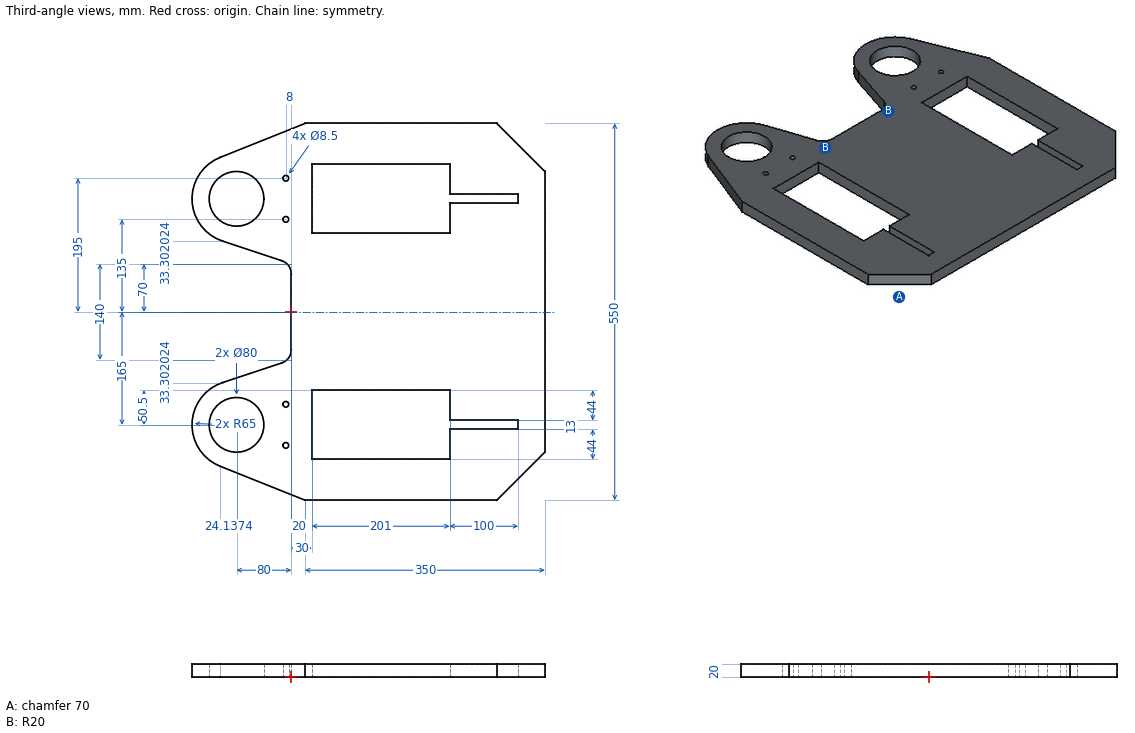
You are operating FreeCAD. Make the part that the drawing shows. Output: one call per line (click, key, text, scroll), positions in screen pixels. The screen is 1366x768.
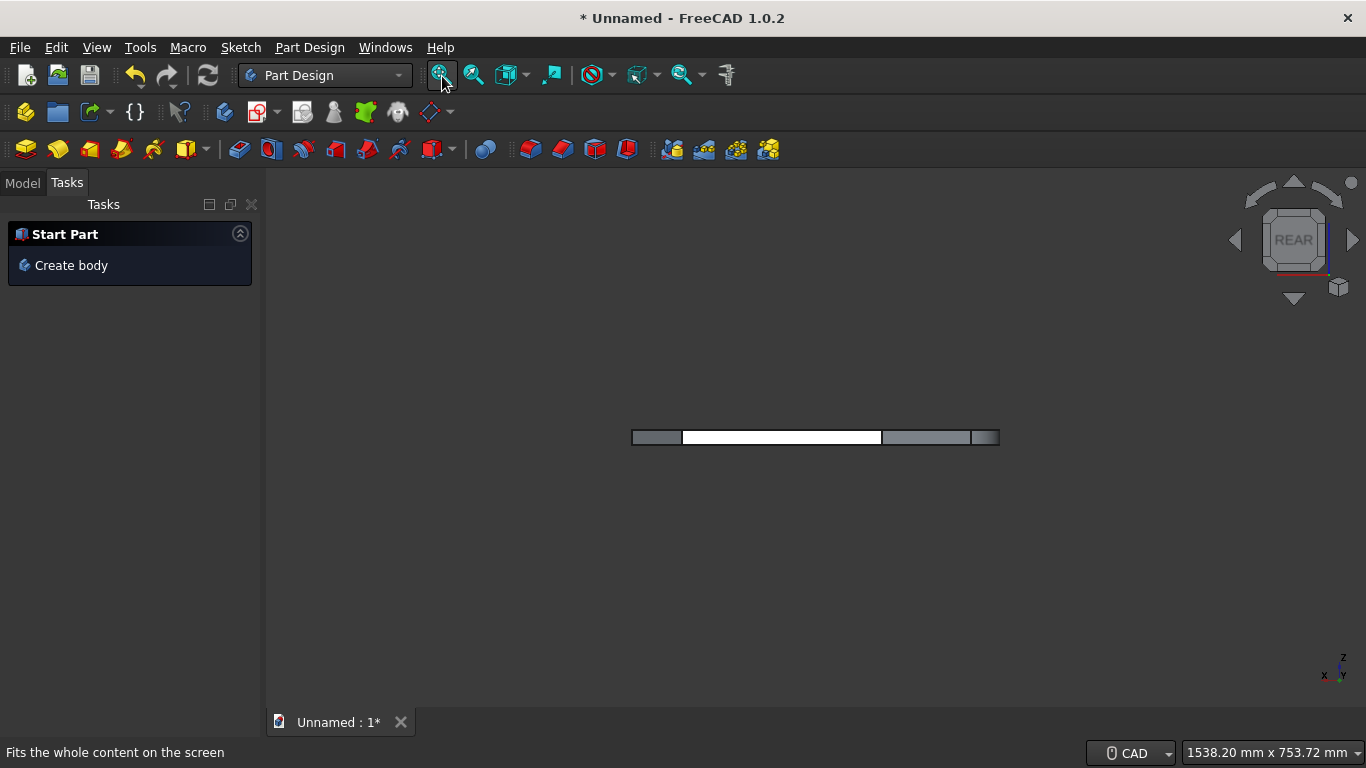
key(6)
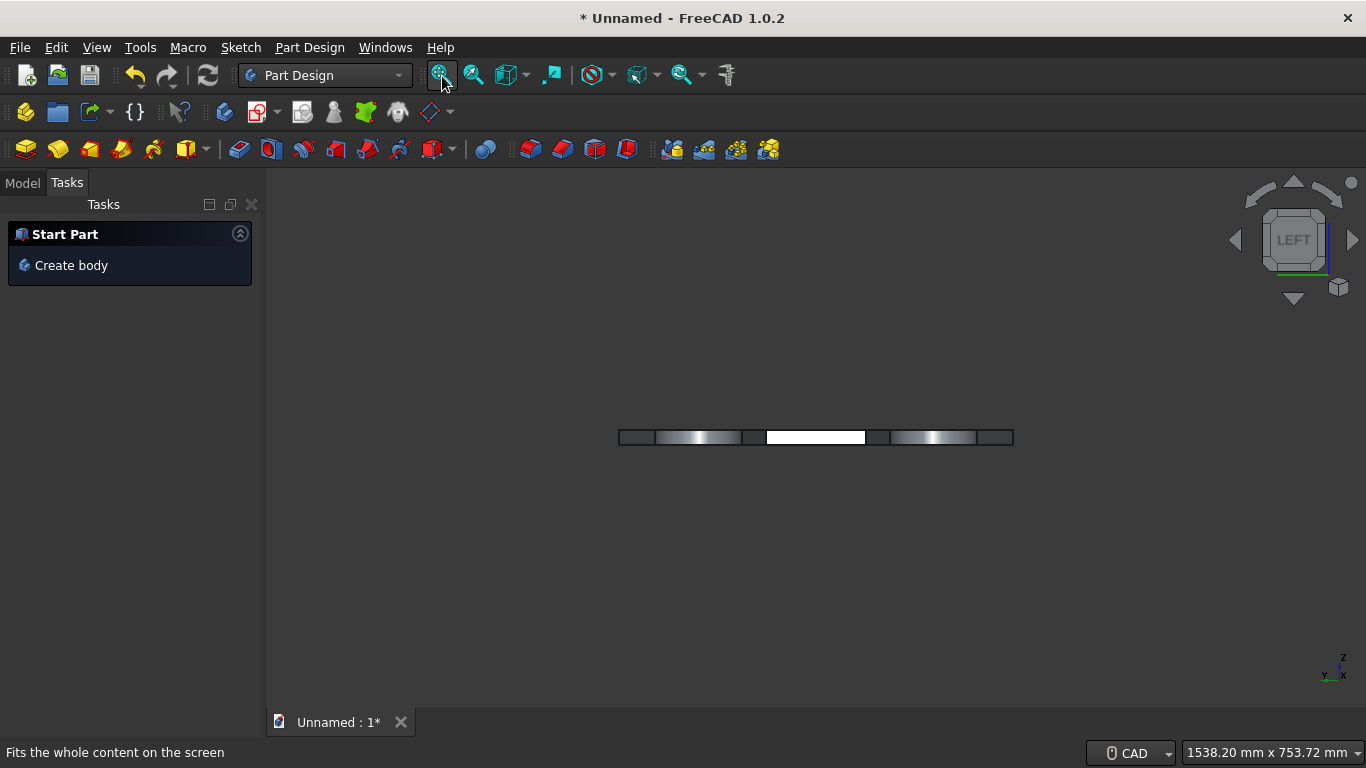
key(v)
key(f)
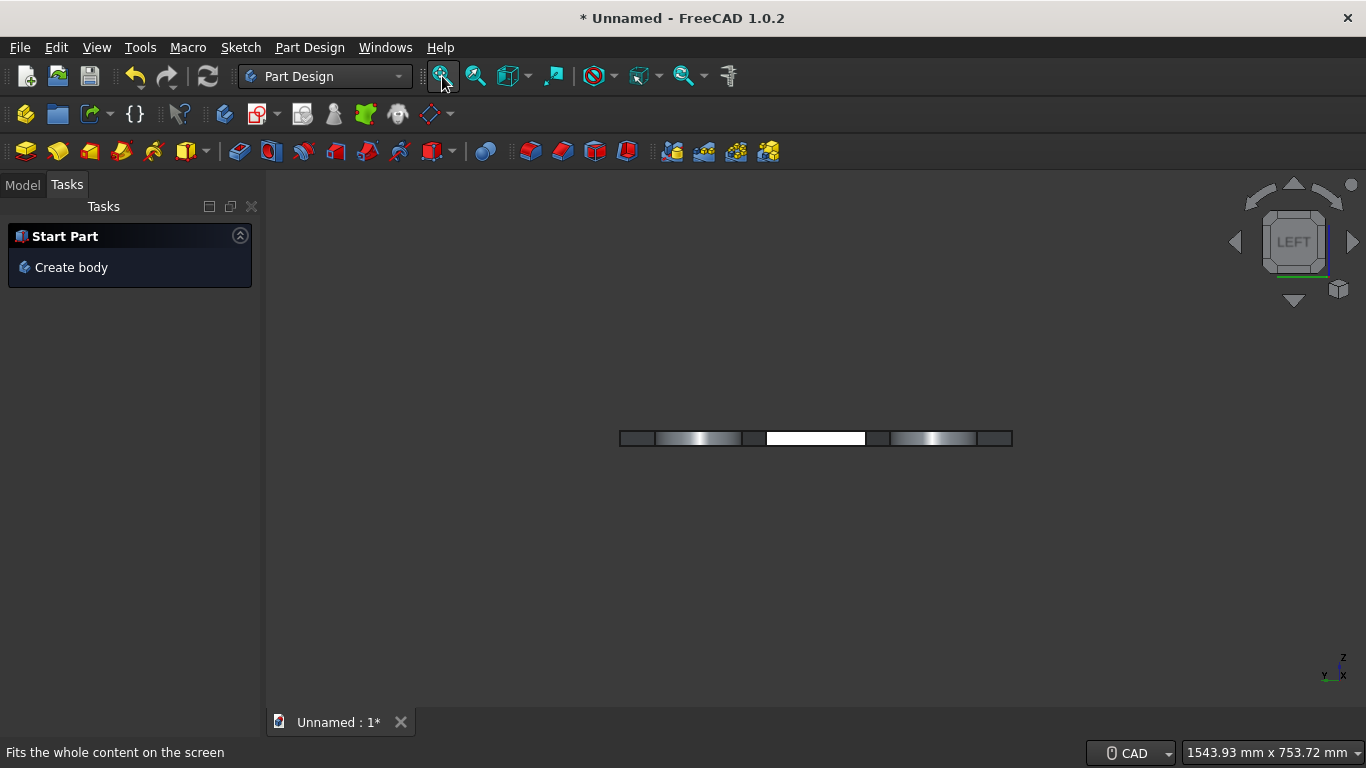
scroll(866, 437, up, 6)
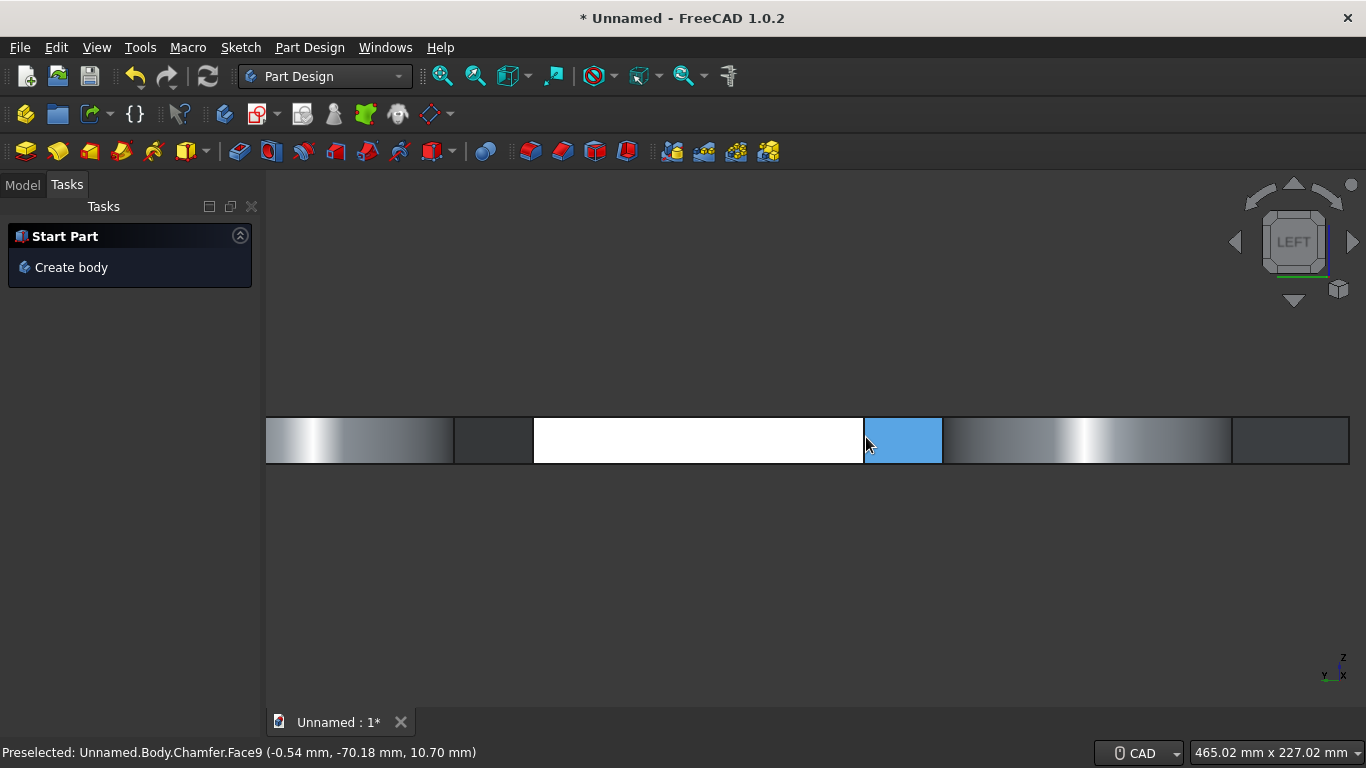
key(v)
key(f)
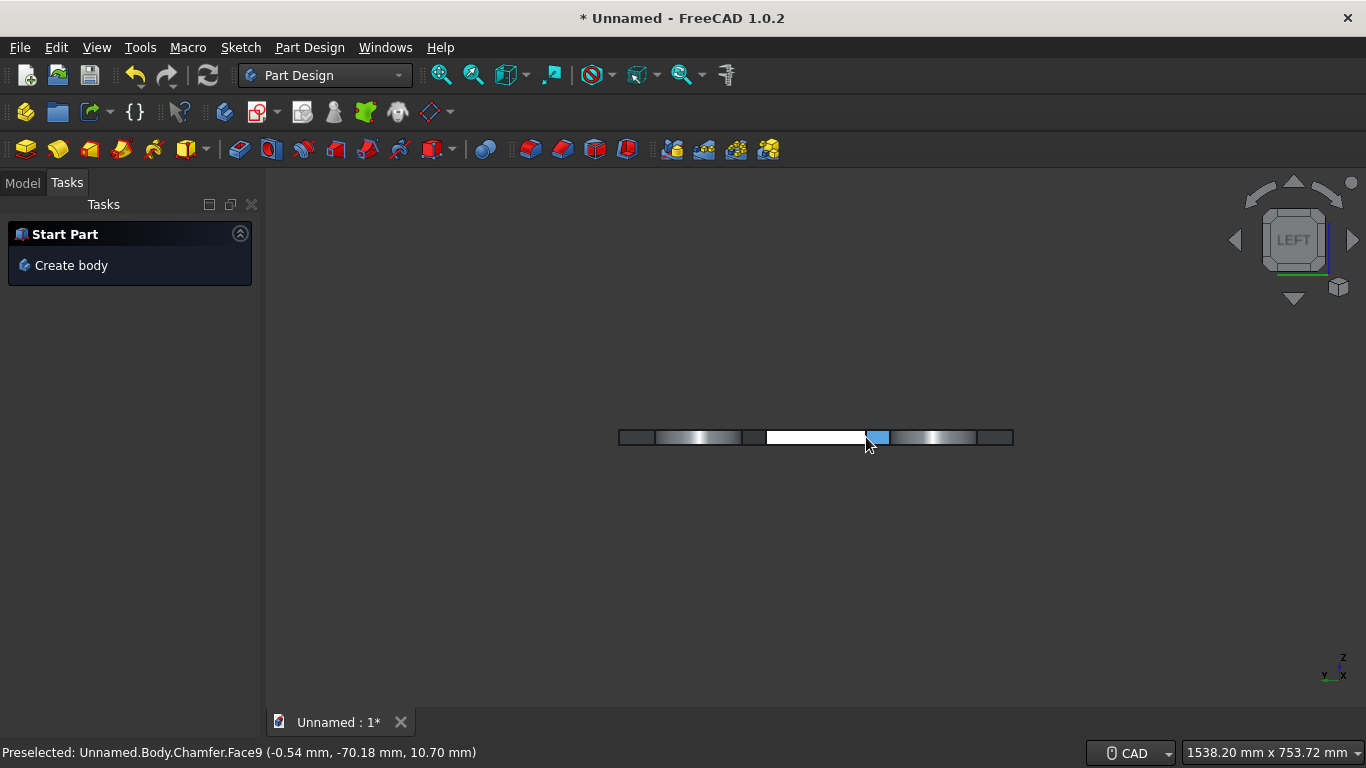
key(v)
key(3)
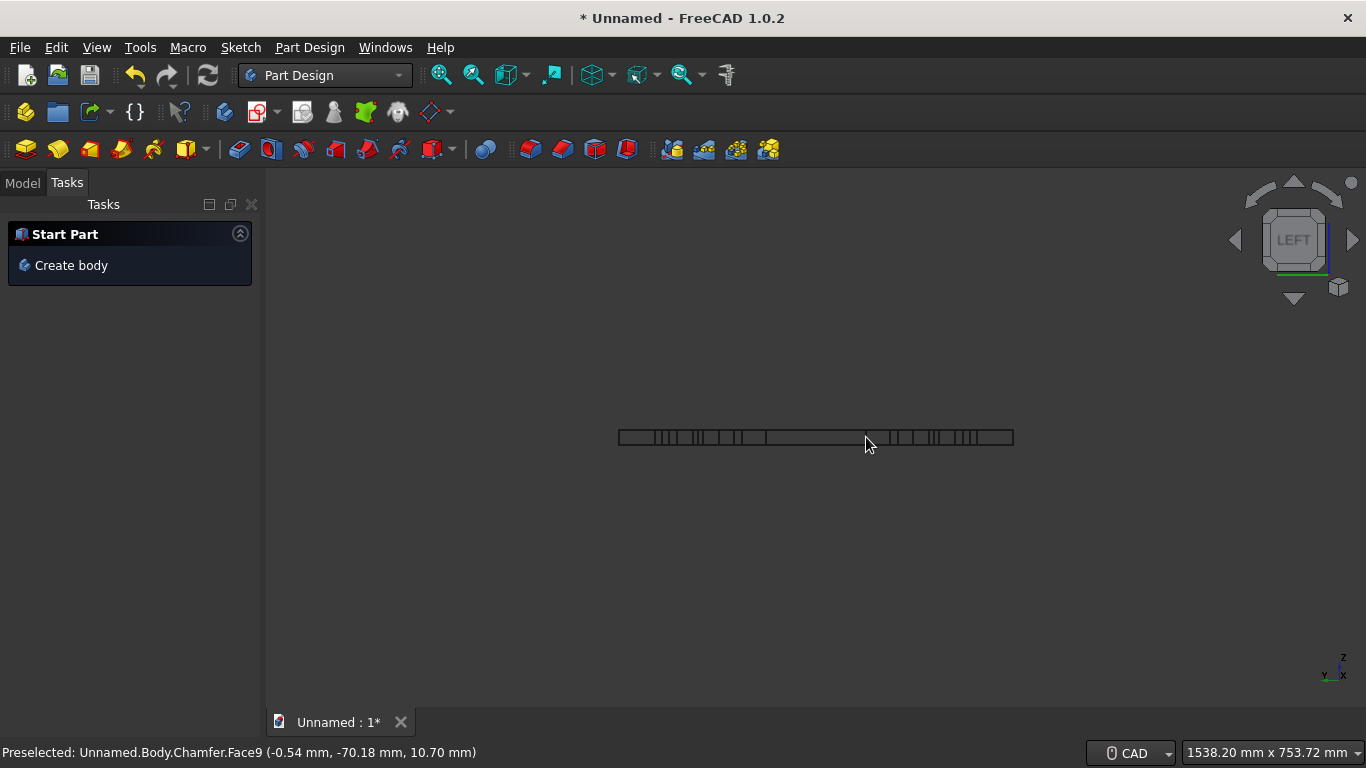
key(0)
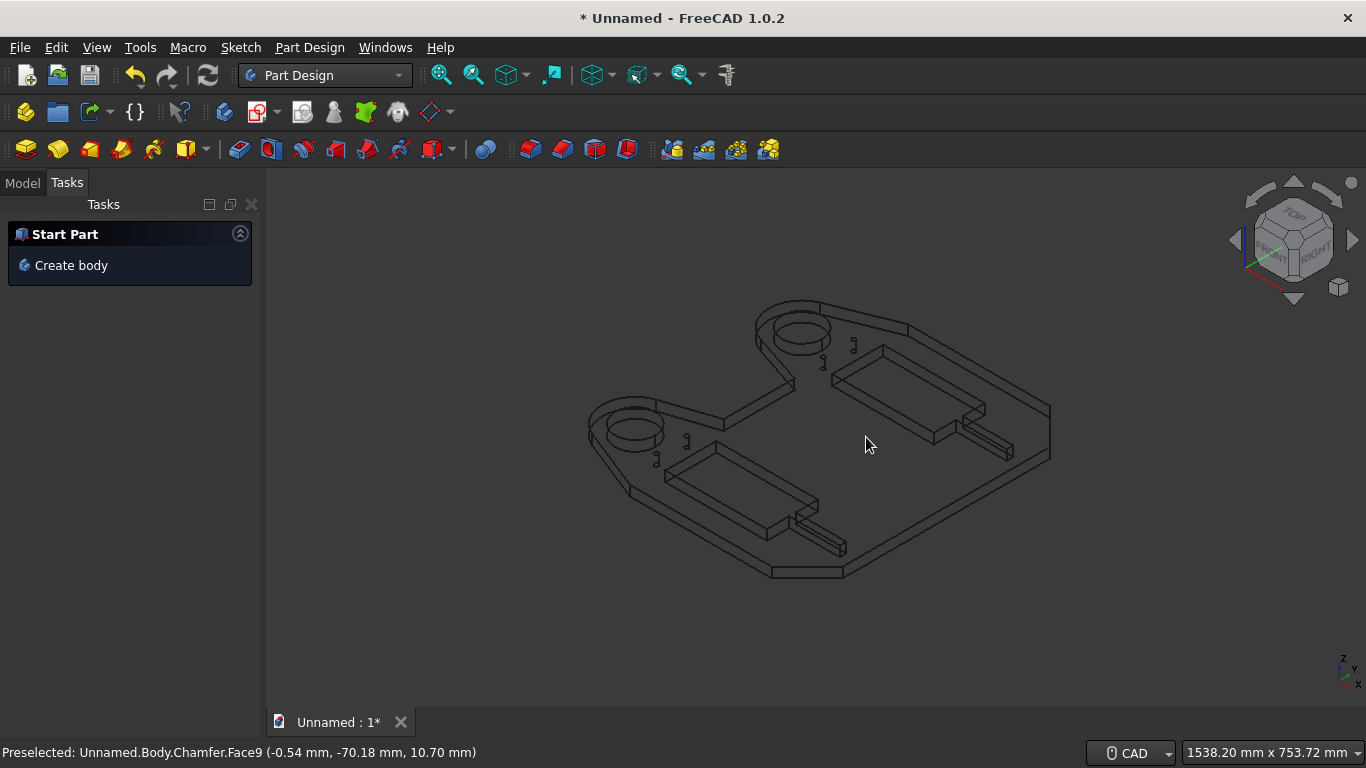
click(724, 425)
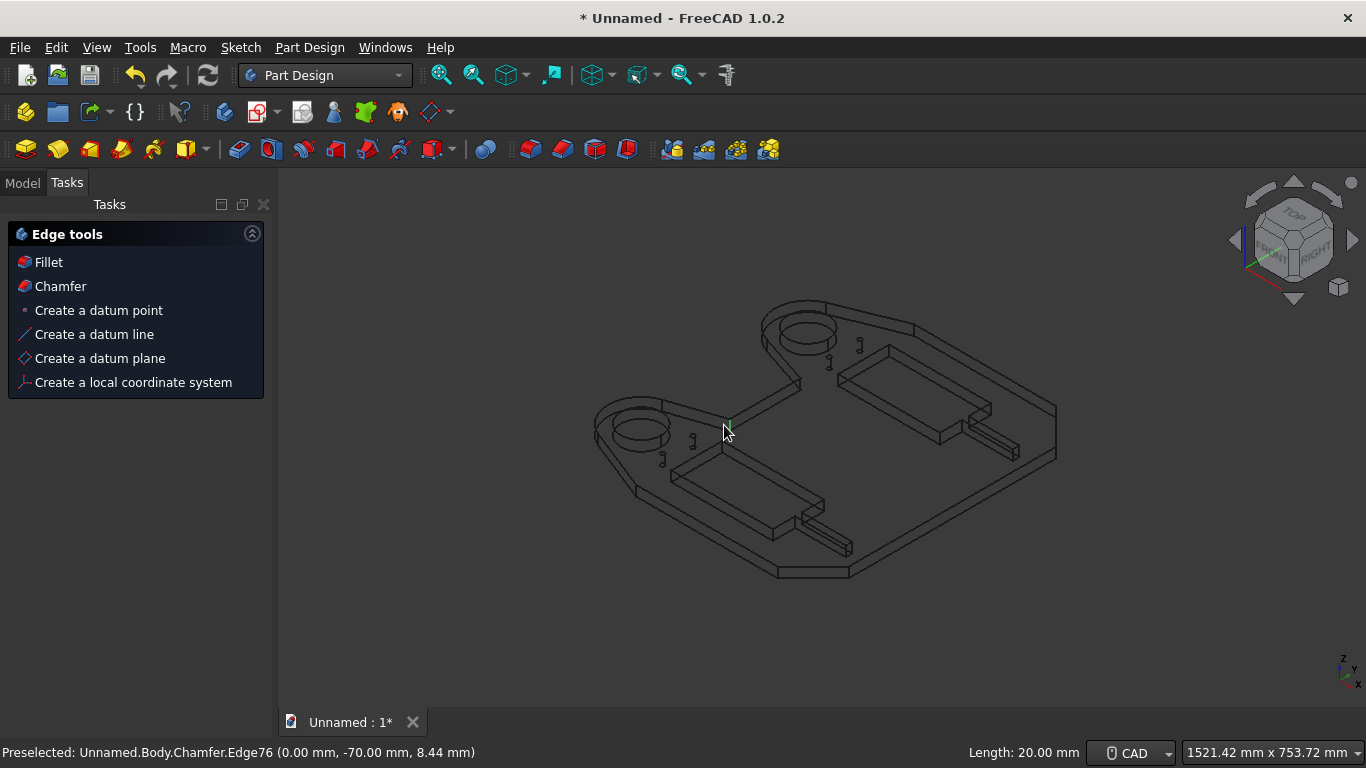
click(801, 386, ctrl)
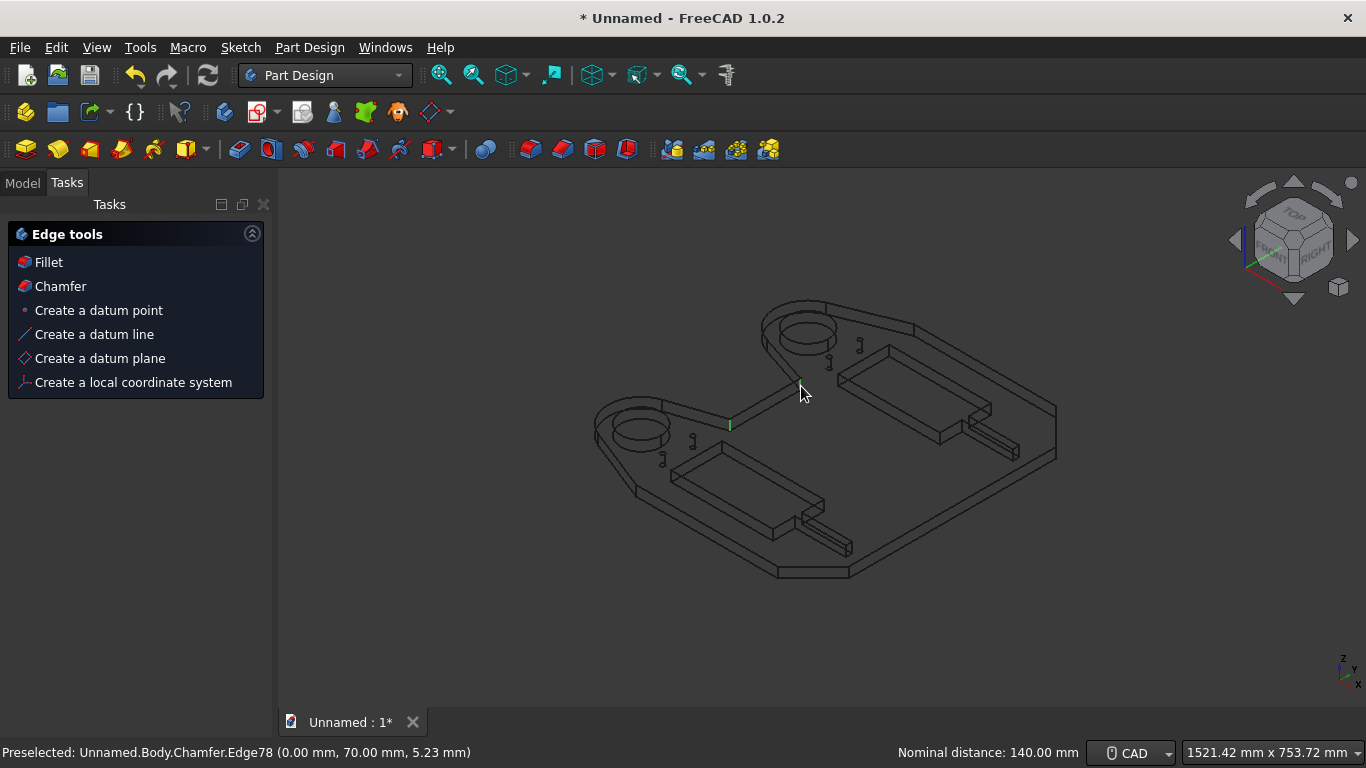
key(v)
key(1)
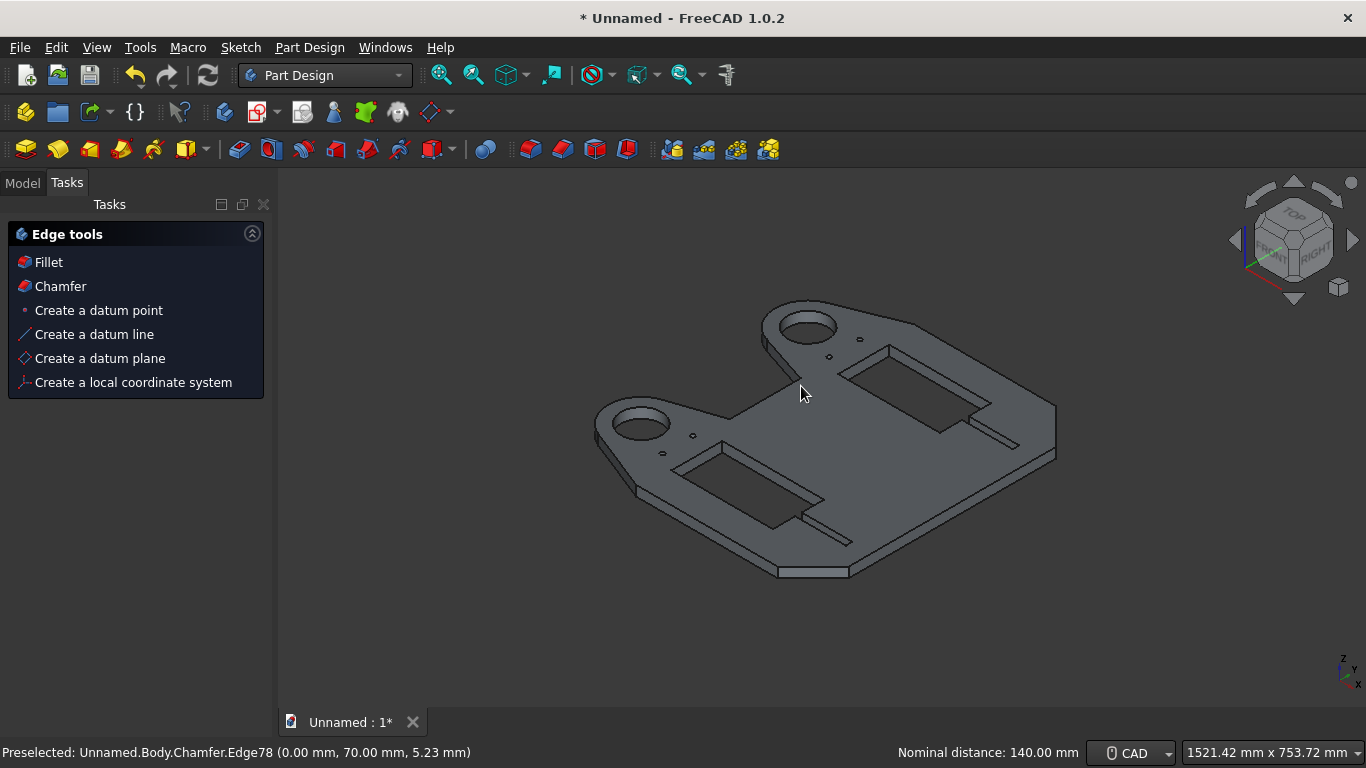
click(532, 150)